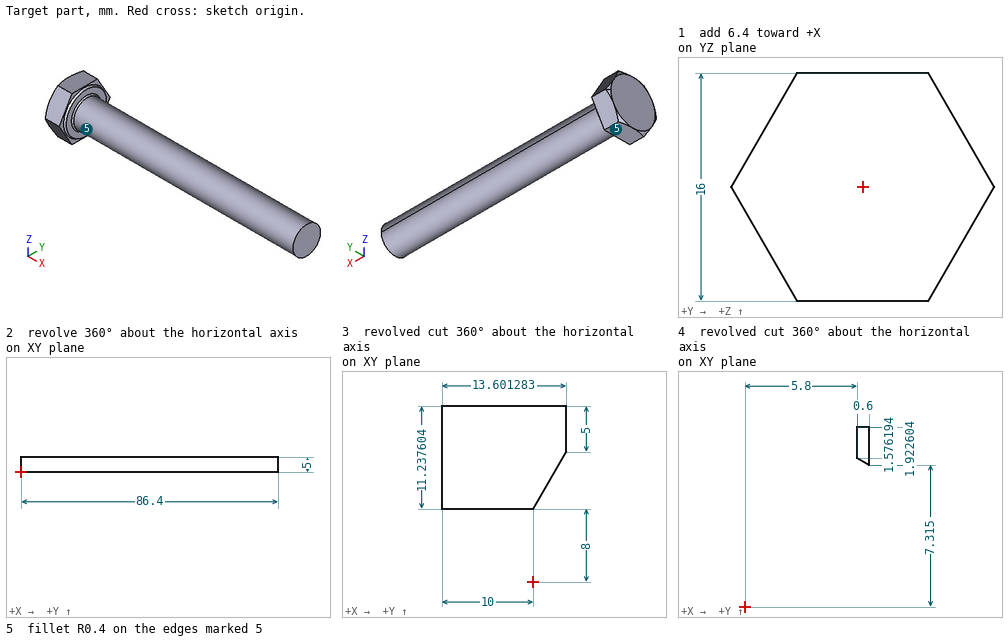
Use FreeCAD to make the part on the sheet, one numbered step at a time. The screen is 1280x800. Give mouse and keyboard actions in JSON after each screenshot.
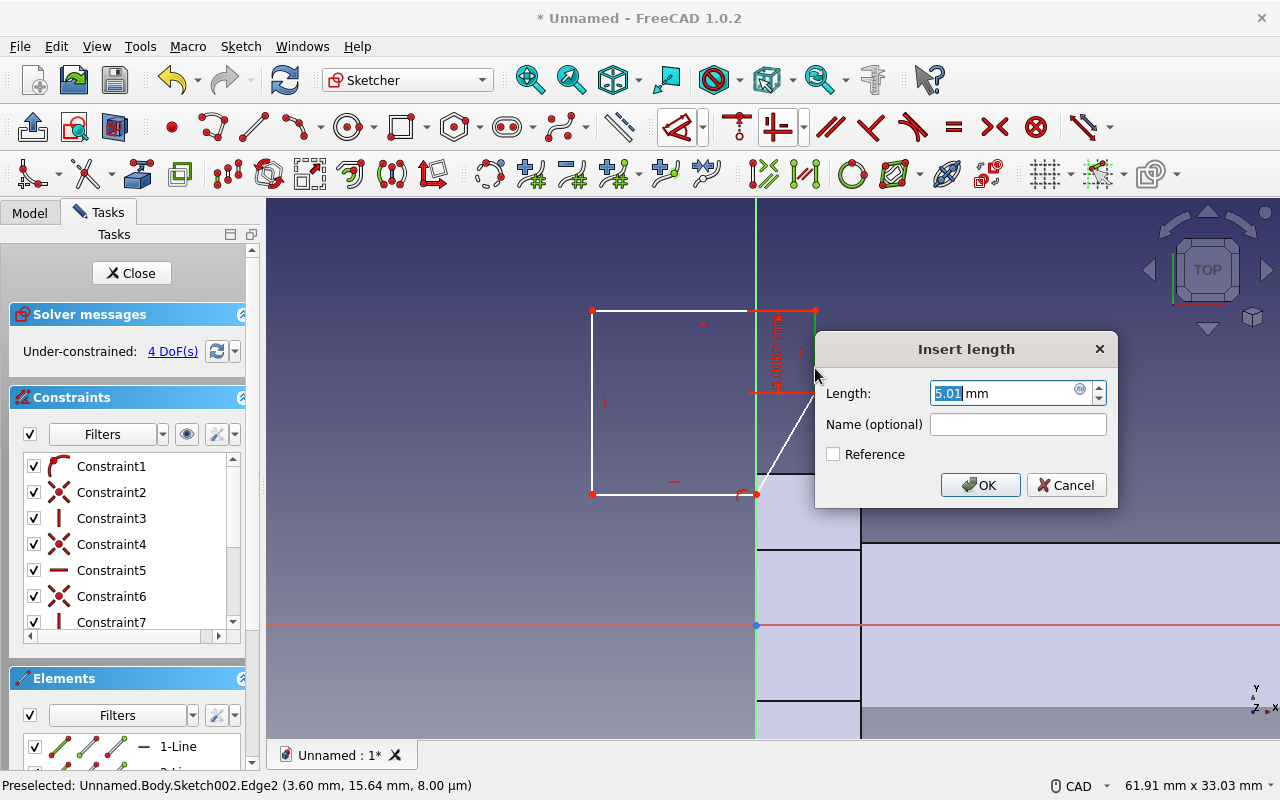
{"action": "type", "text": "5"}
{"action": "key", "text": "Return"}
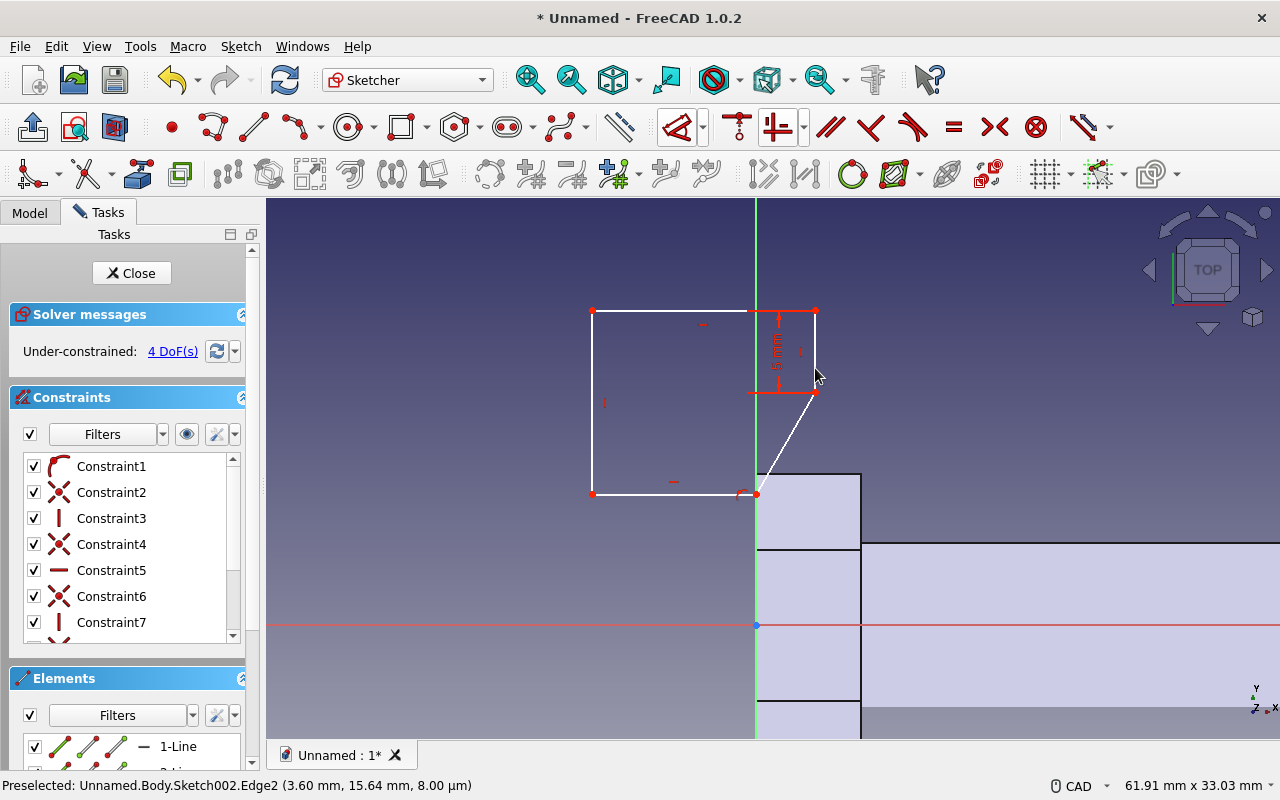
{"action": "left_click", "coordinate": [641, 495]}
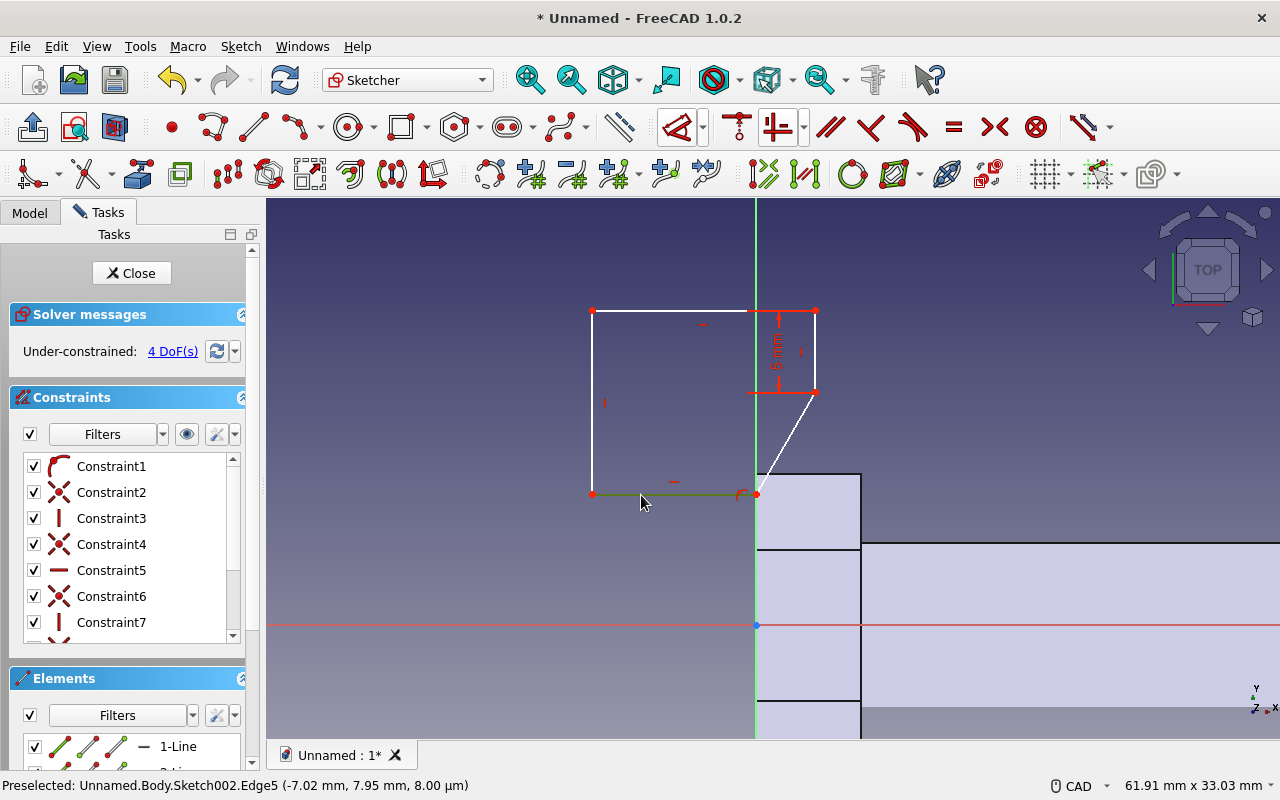
{"action": "key", "text": "l"}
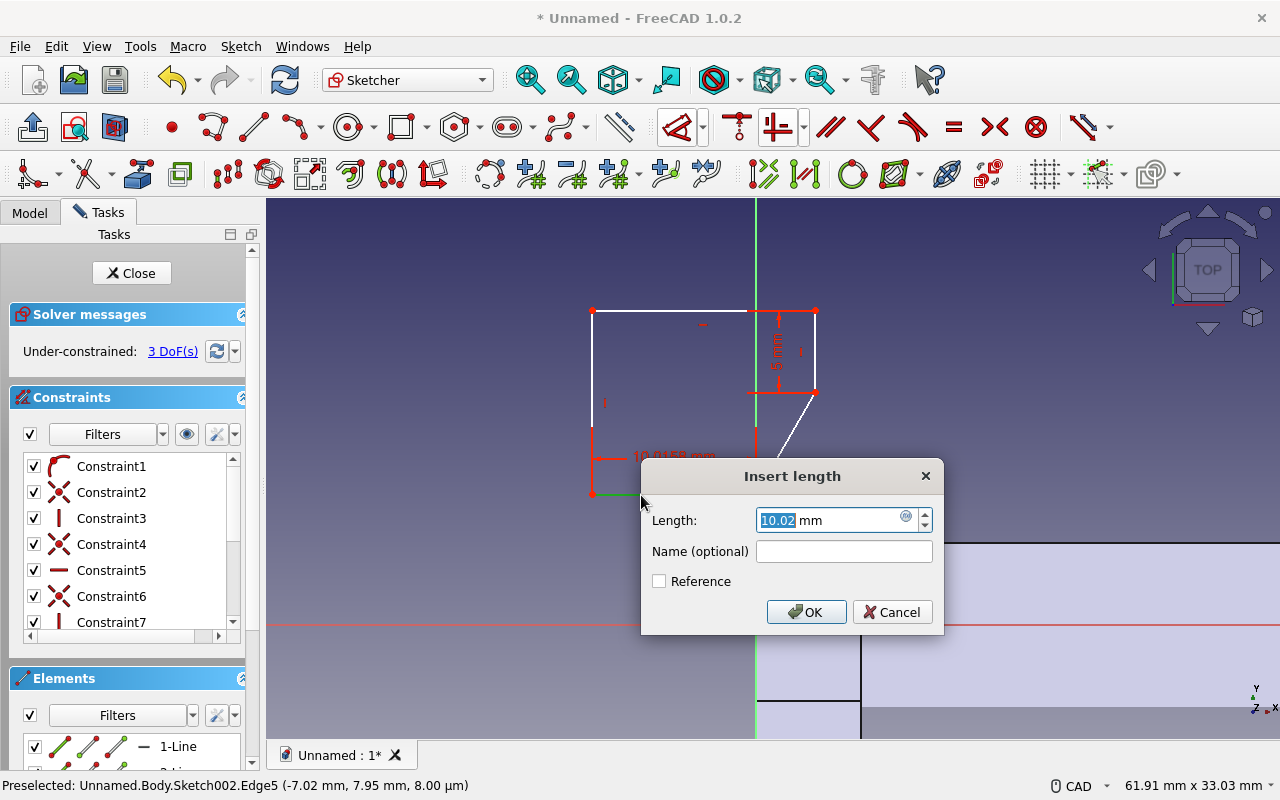
{"action": "type", "text": "10"}
{"action": "key", "text": "Return"}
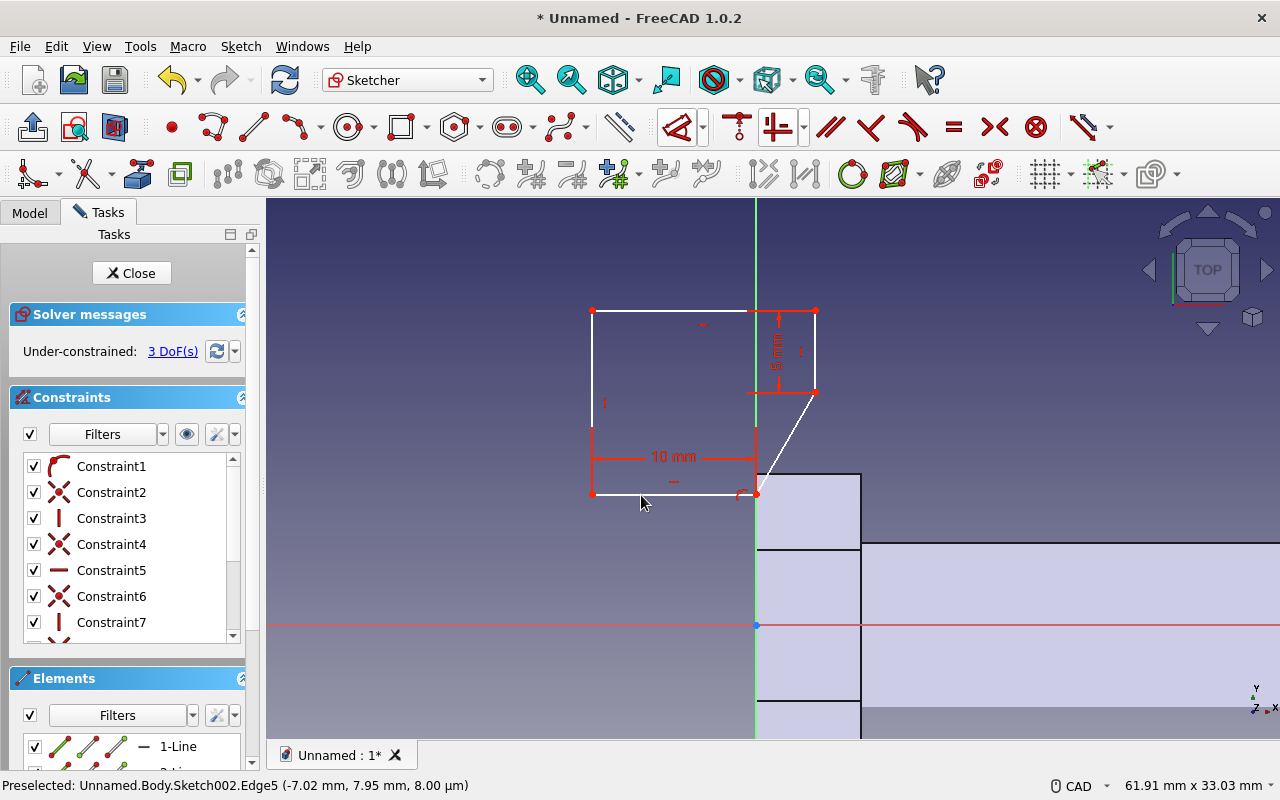
{"action": "left_click", "coordinate": [756, 495]}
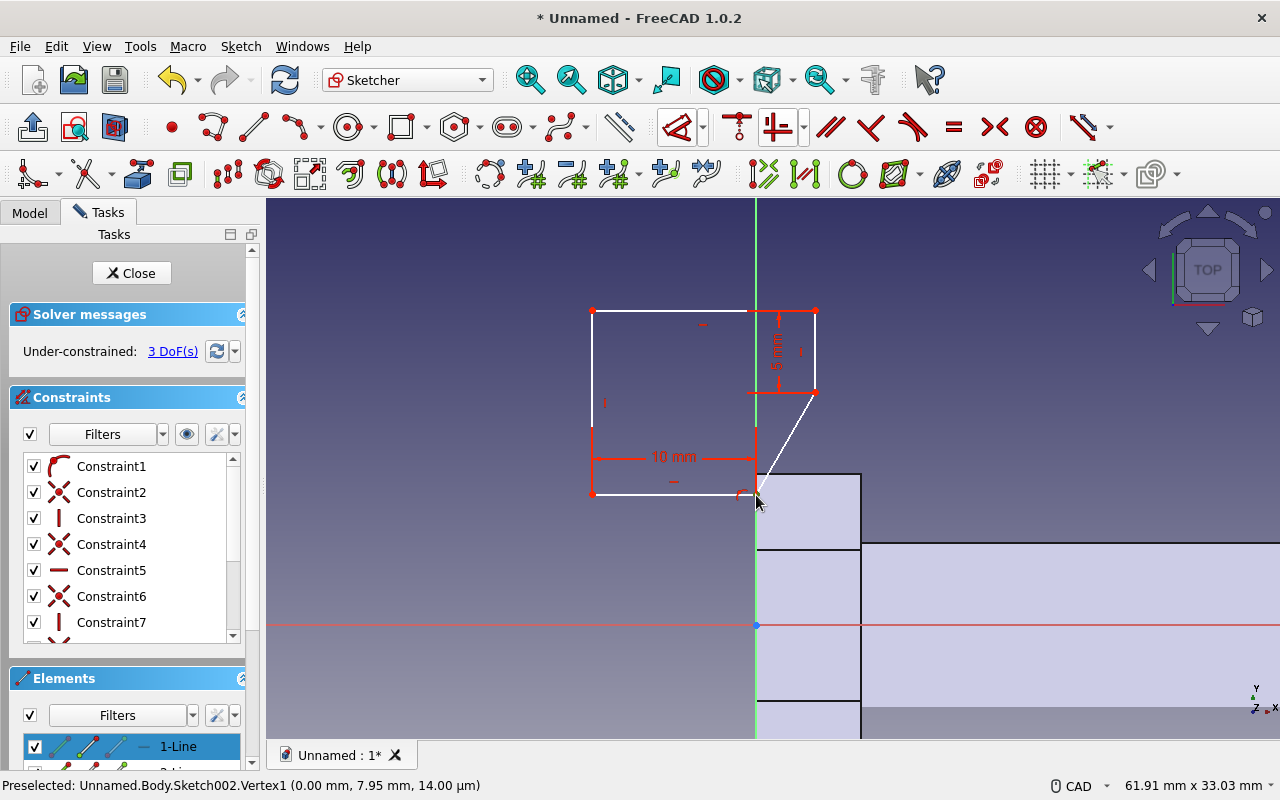
{"action": "left_click", "coordinate": [702, 128]}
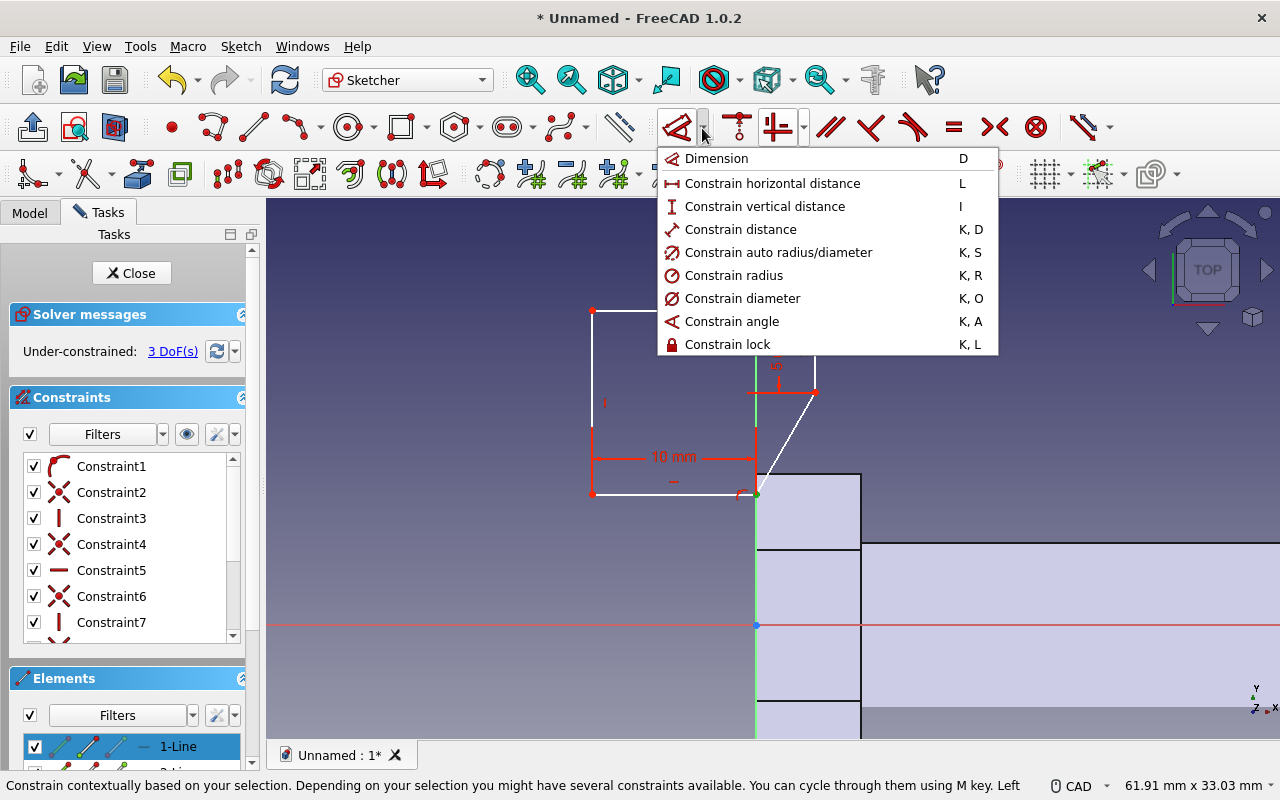
{"action": "left_click", "coordinate": [828, 206]}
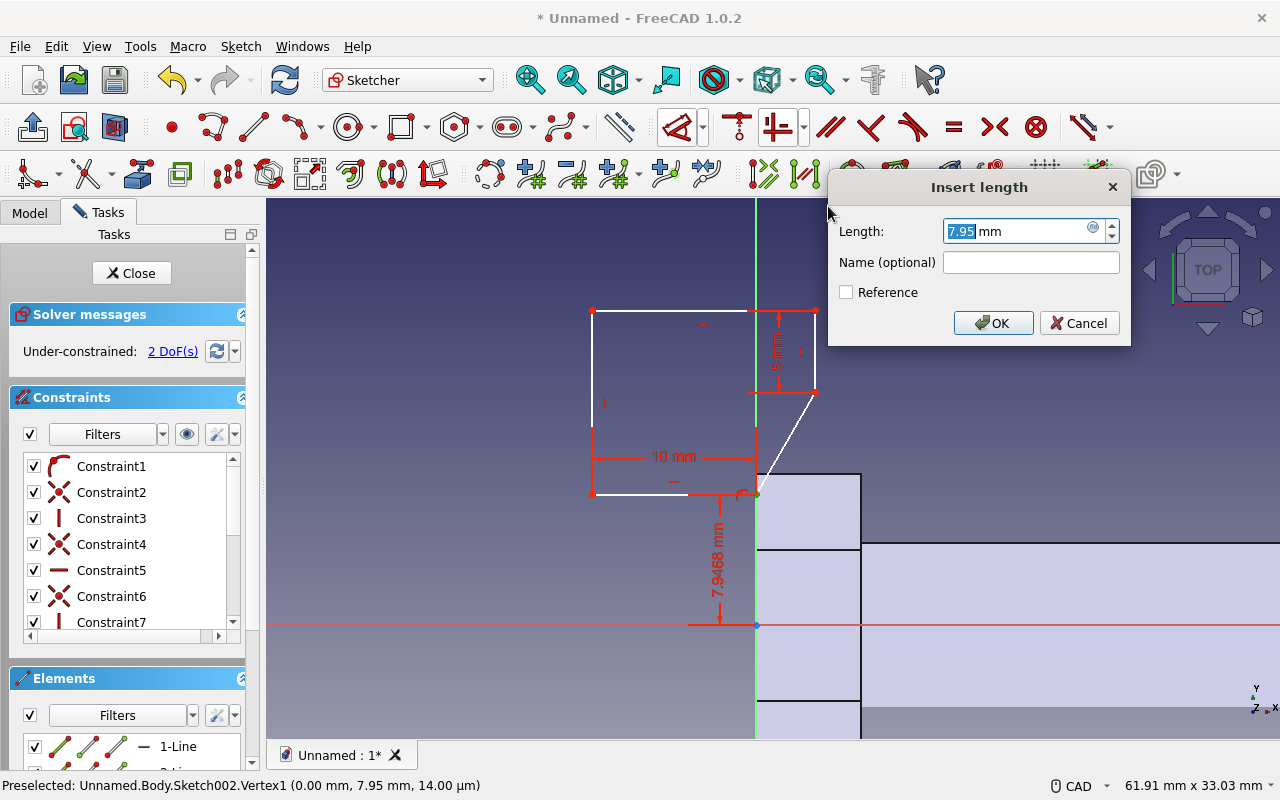
{"action": "type", "text": "8"}
{"action": "key", "text": "Return"}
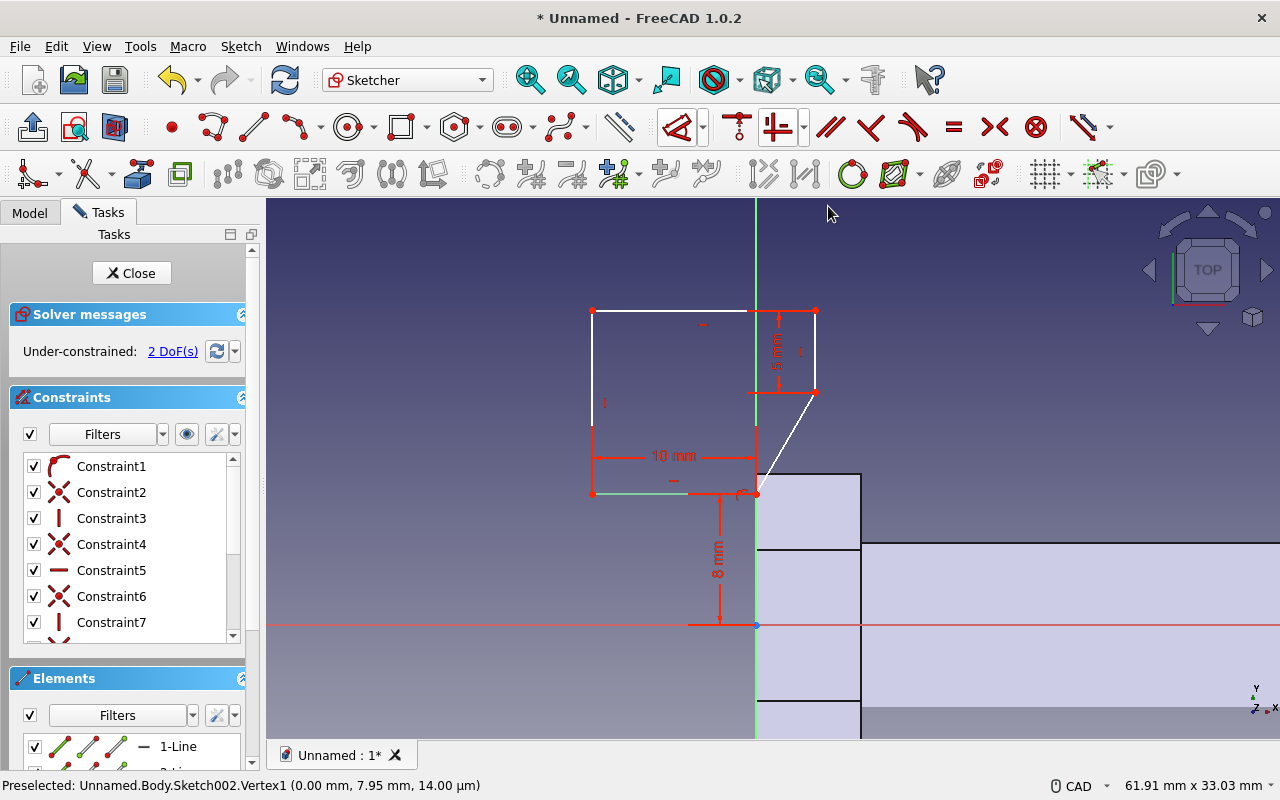
{"action": "left_click", "coordinate": [659, 311]}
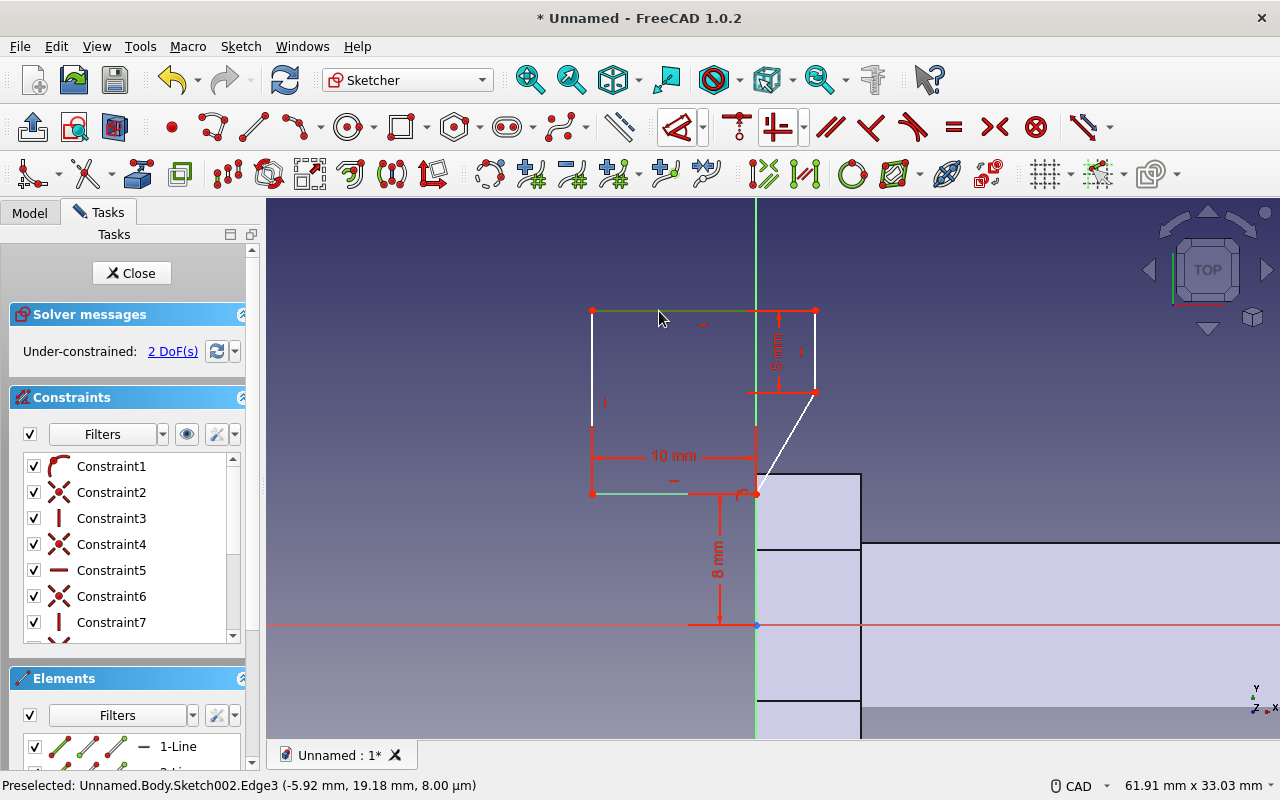
{"action": "key", "text": "l"}